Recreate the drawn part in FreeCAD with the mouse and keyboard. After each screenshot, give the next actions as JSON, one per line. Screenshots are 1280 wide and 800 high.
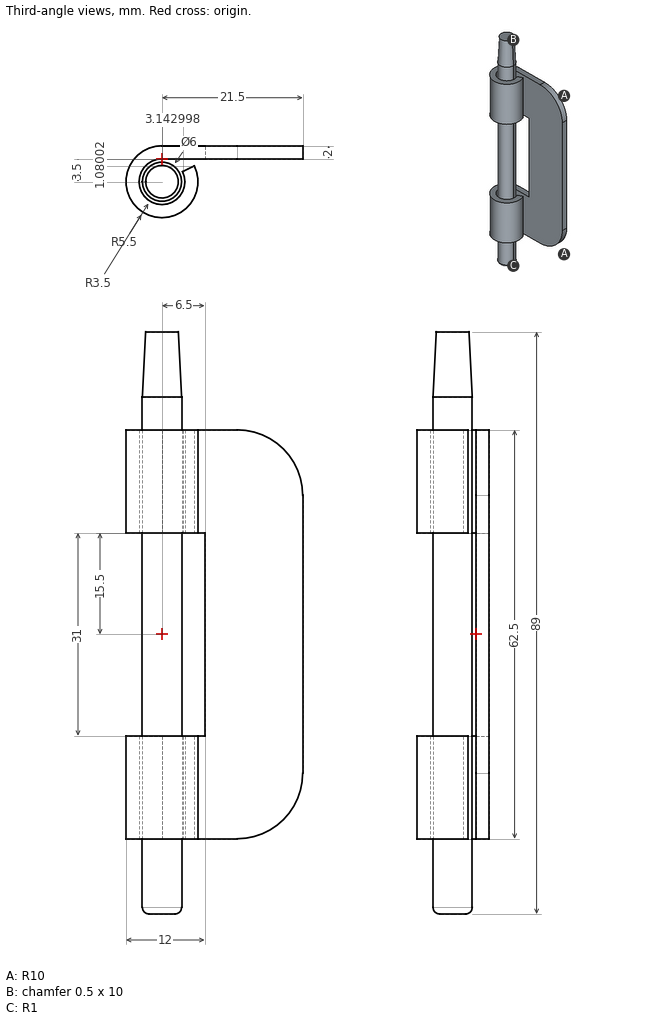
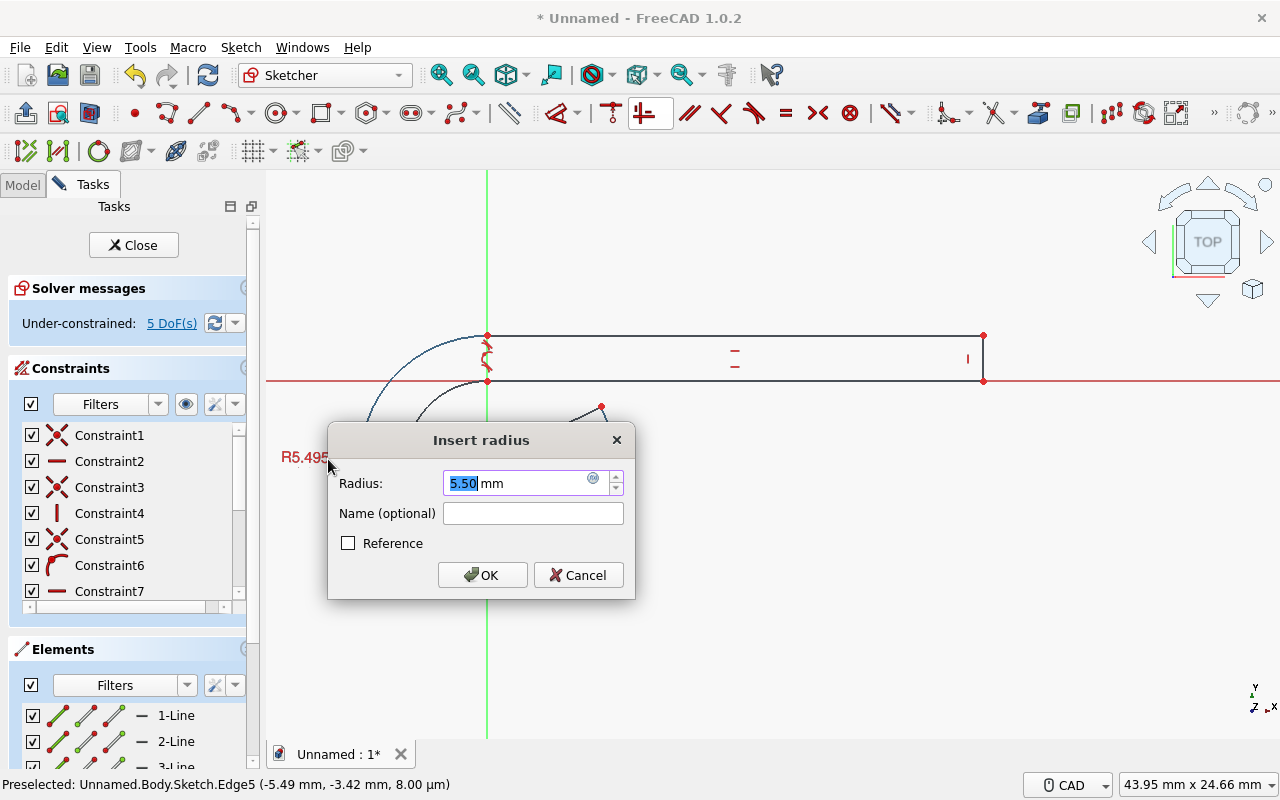
{"action": "type", "text": "5.5"}
{"action": "key", "text": "Return"}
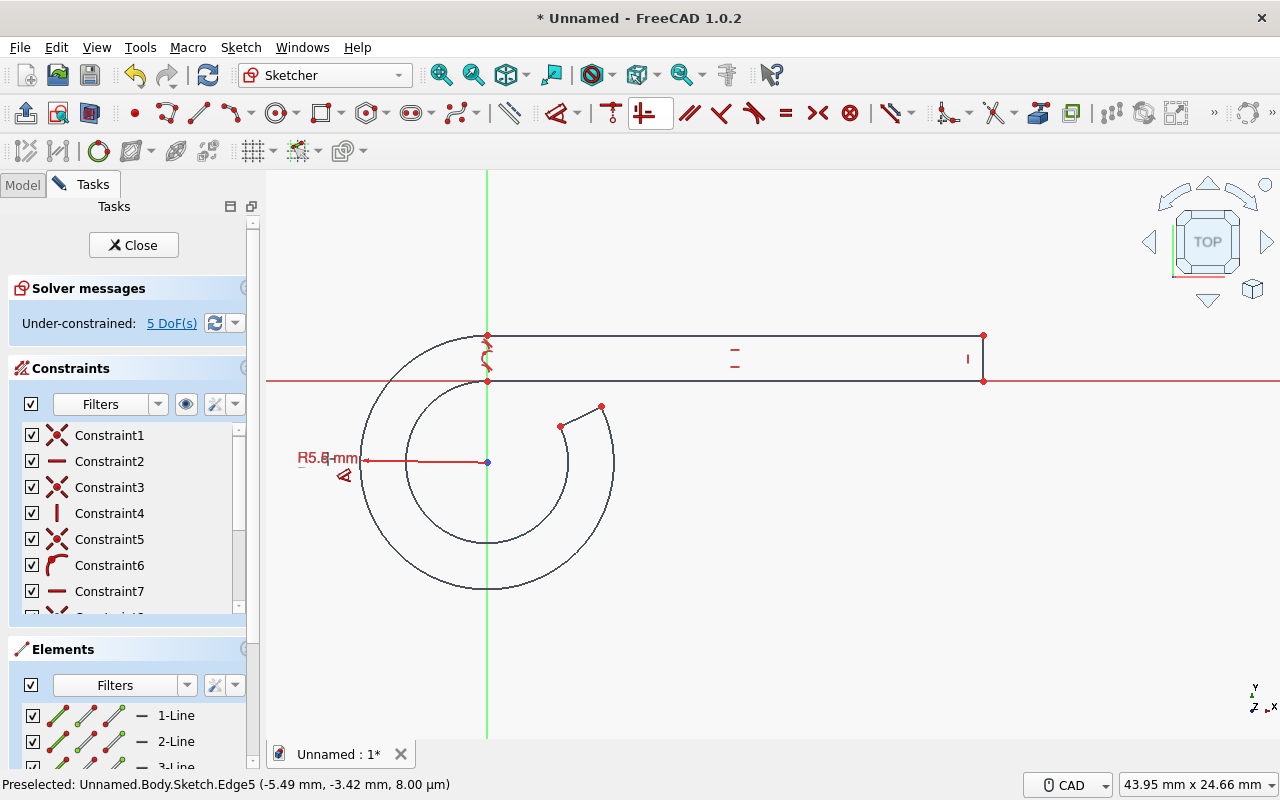
{"action": "left_click", "coordinate": [406, 460]}
{"action": "left_click", "coordinate": [389, 405]}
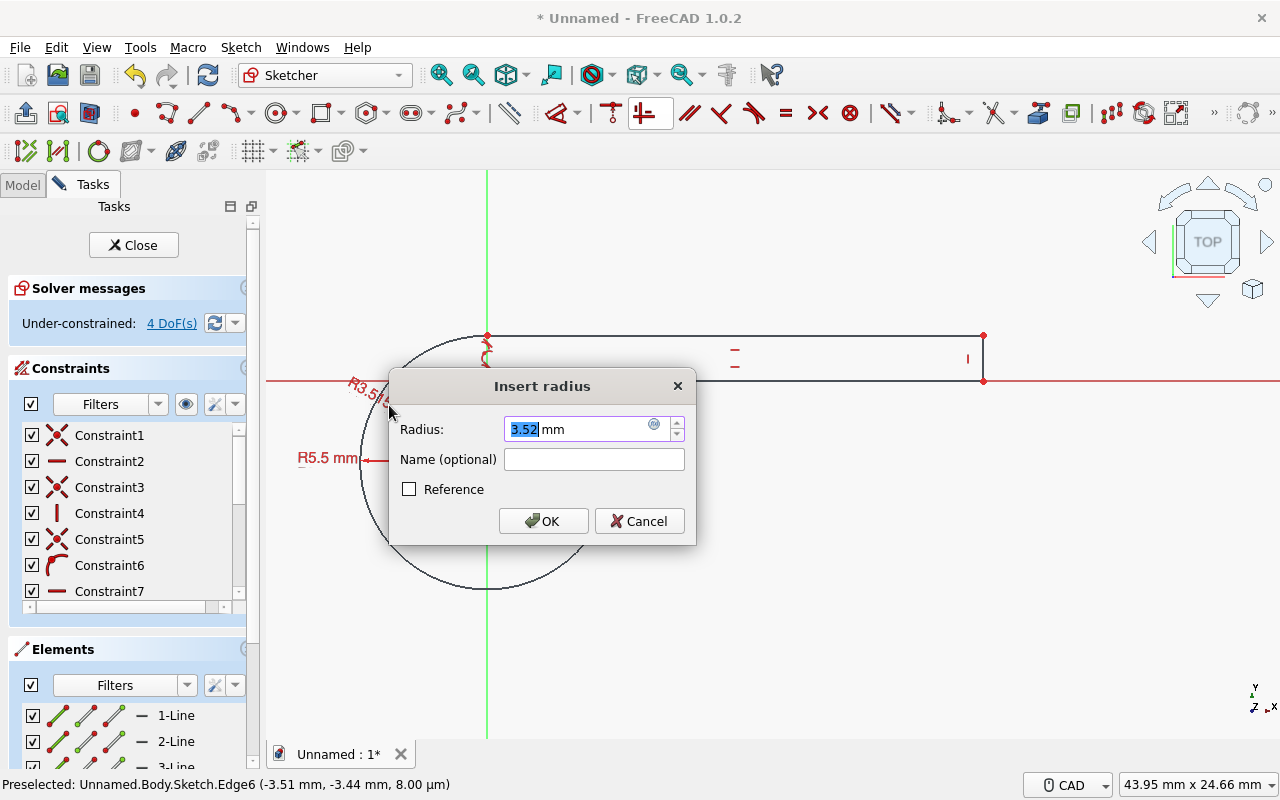
{"action": "type", "text": "3.5"}
{"action": "key", "text": "Return"}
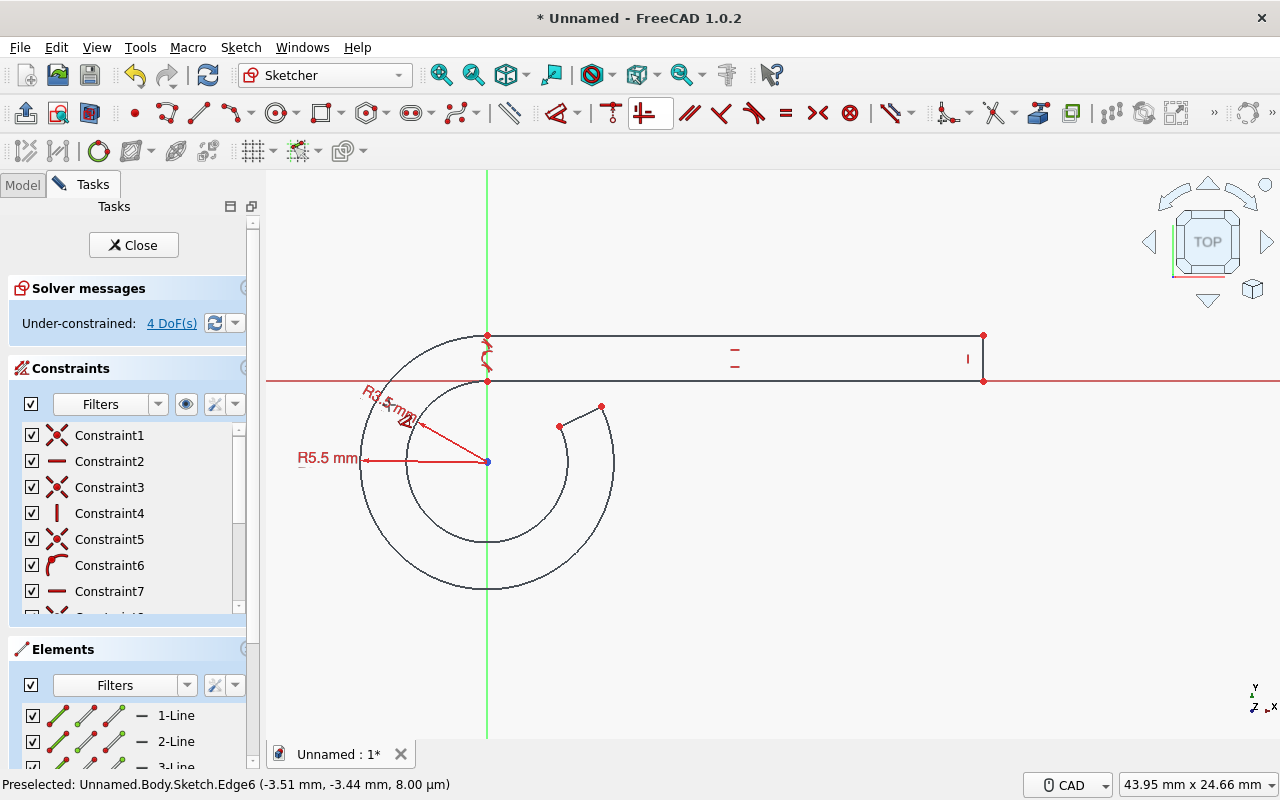
{"action": "left_click", "coordinate": [983, 367]}
{"action": "left_click", "coordinate": [1017, 358]}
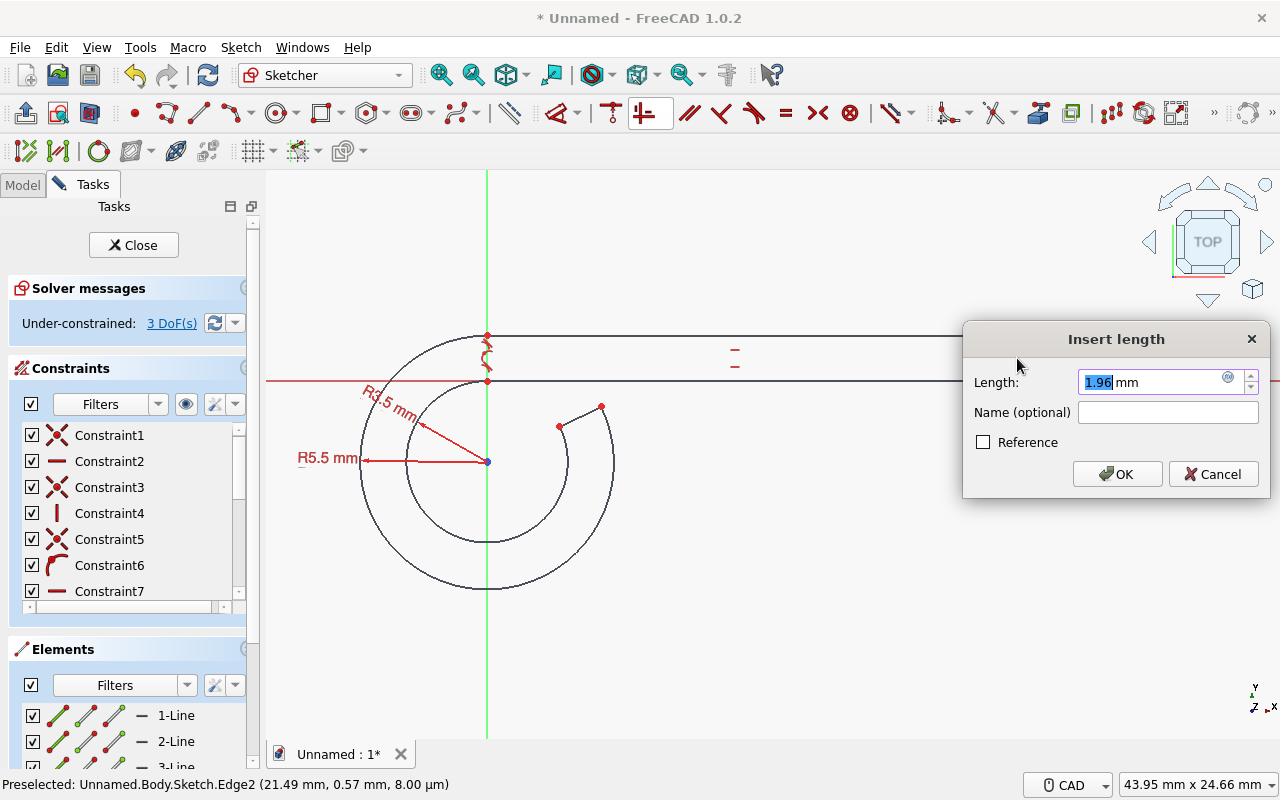
{"action": "type", "text": "2"}
{"action": "key", "text": "Return"}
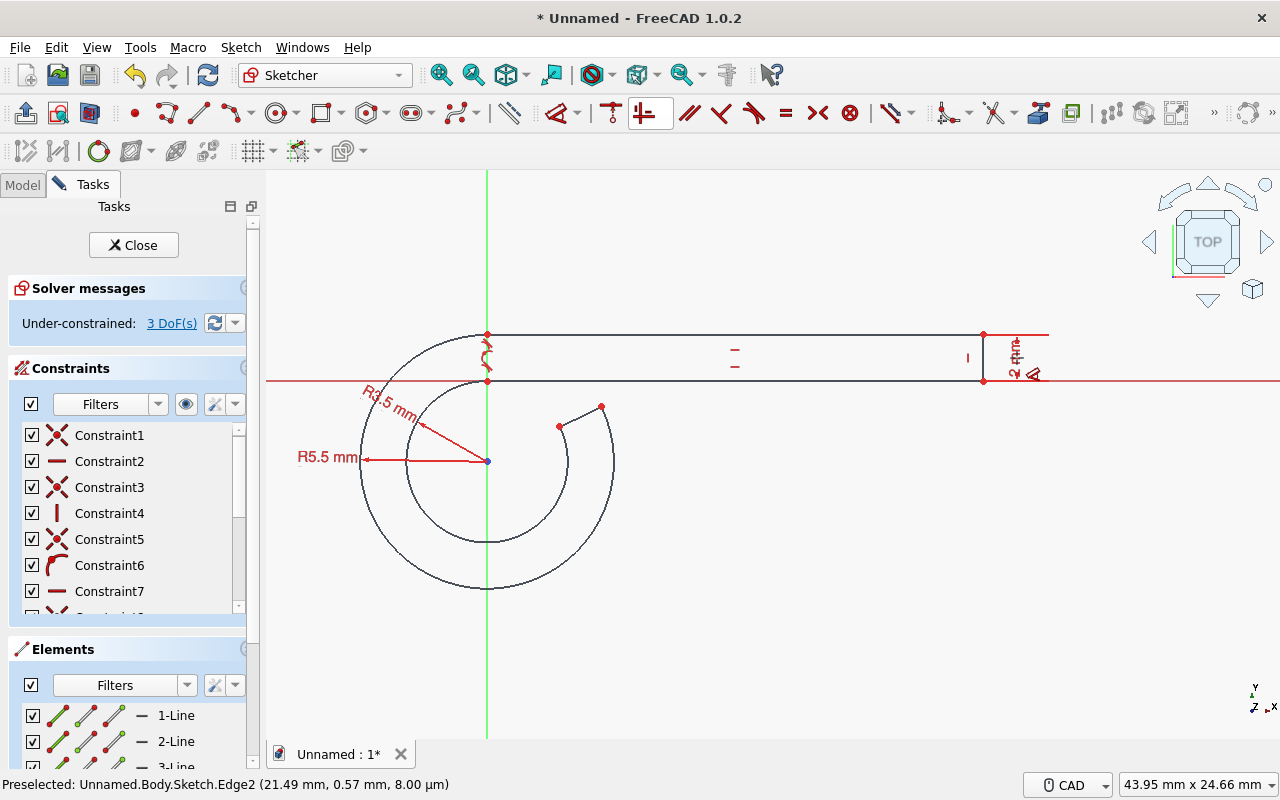
{"action": "left_click", "coordinate": [636, 381]}
{"action": "left_click", "coordinate": [735, 415]}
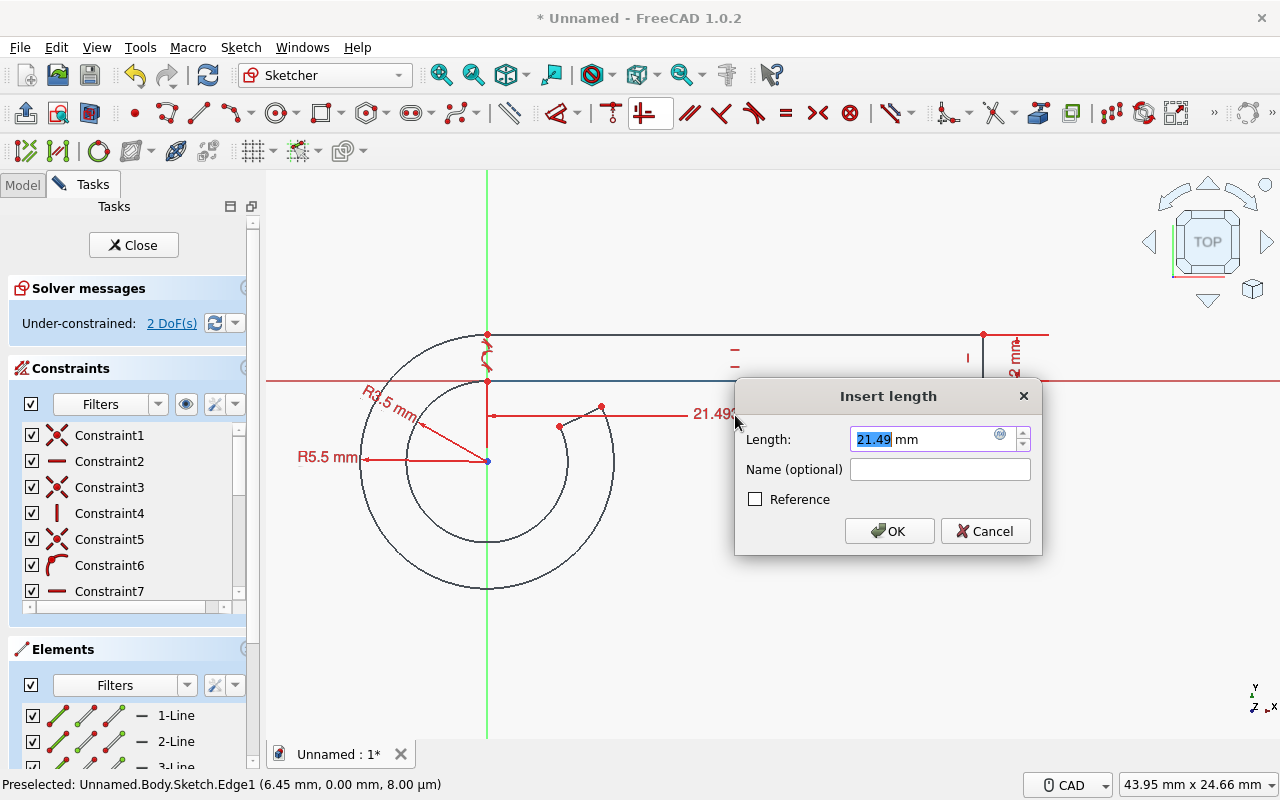
{"action": "type", "text": "21.5"}
{"action": "key", "text": "Return"}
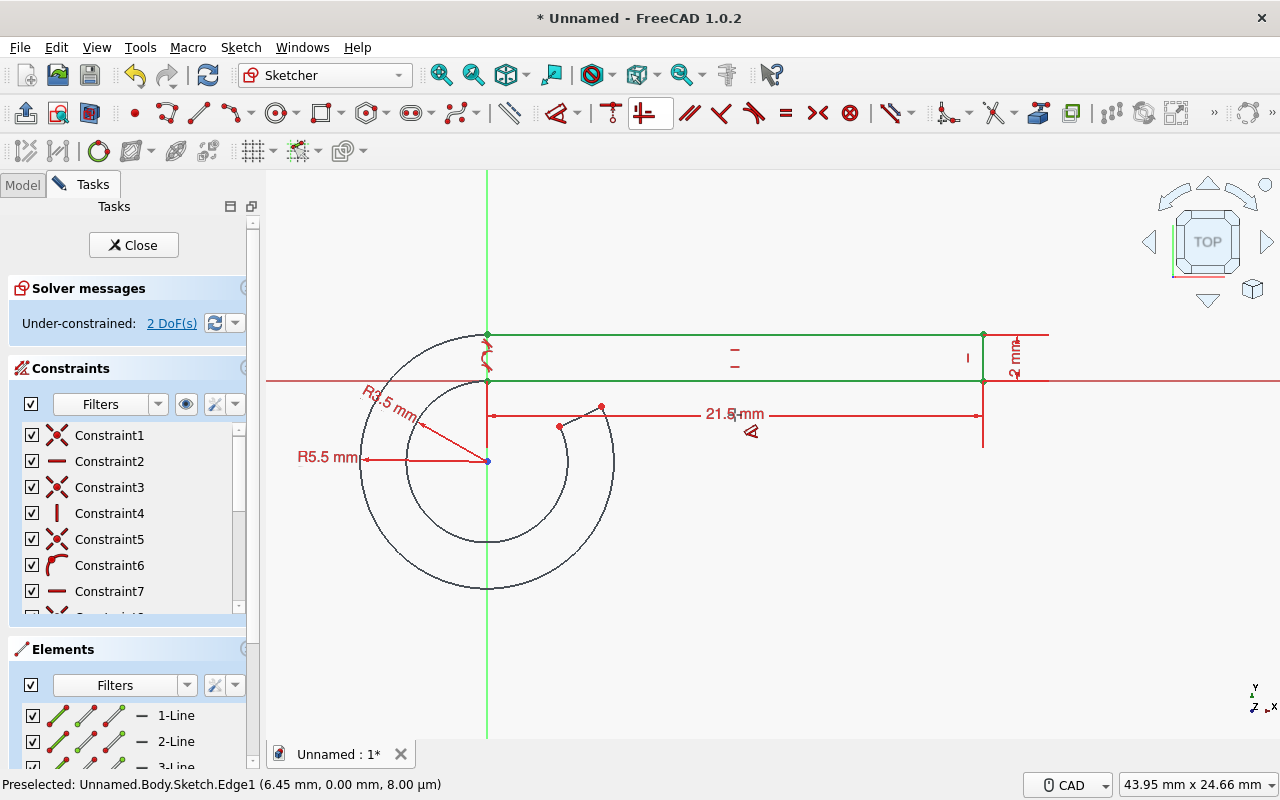
{"action": "scroll", "coordinate": [602, 407], "scroll_direction": "up", "scroll_amount": 3}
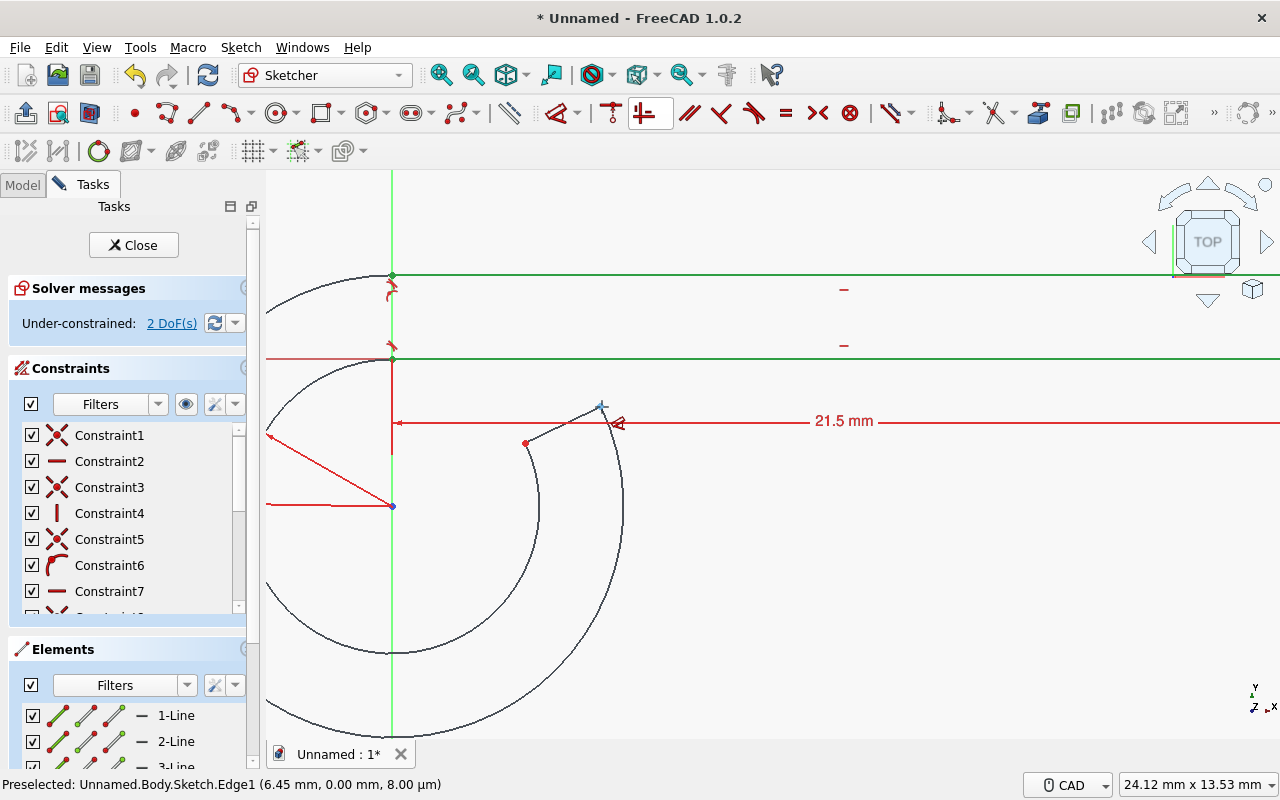
{"action": "left_click", "coordinate": [601, 407]}
{"action": "left_click", "coordinate": [358, 383]}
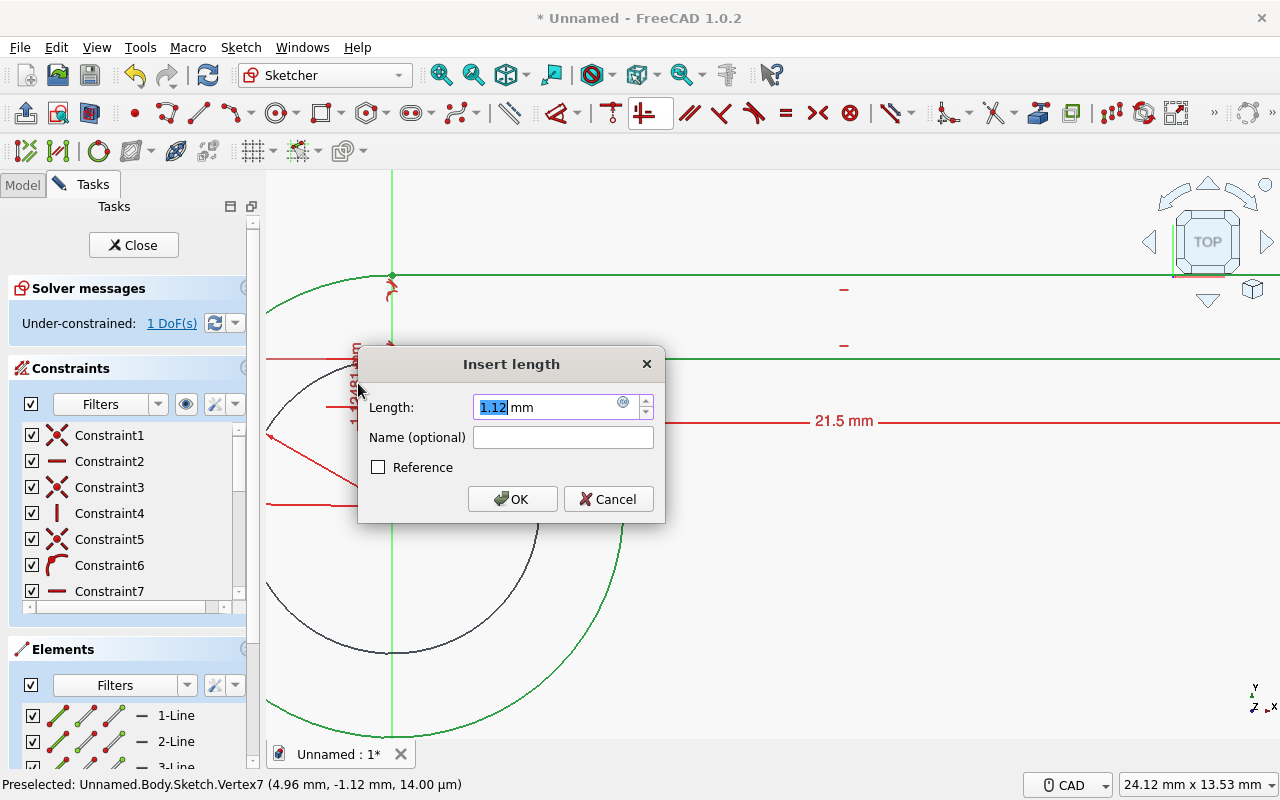
{"action": "type", "text": "1.08002"}
{"action": "key", "text": "Return"}